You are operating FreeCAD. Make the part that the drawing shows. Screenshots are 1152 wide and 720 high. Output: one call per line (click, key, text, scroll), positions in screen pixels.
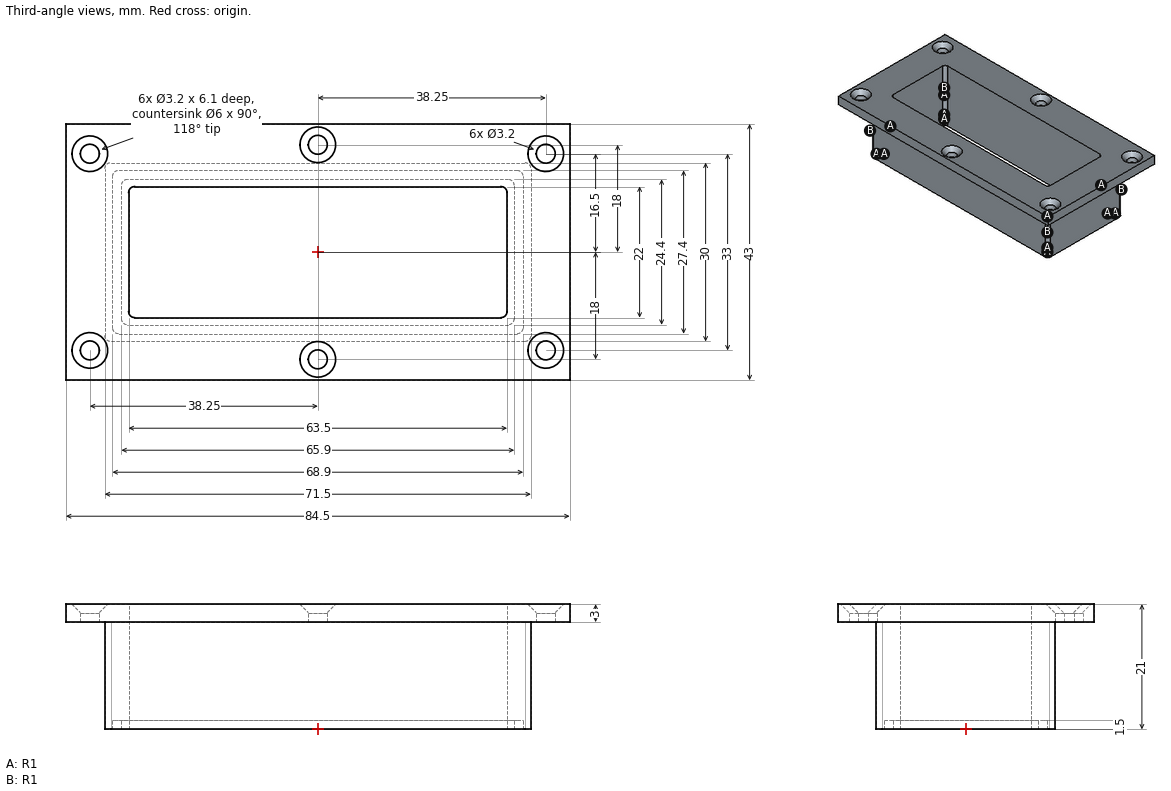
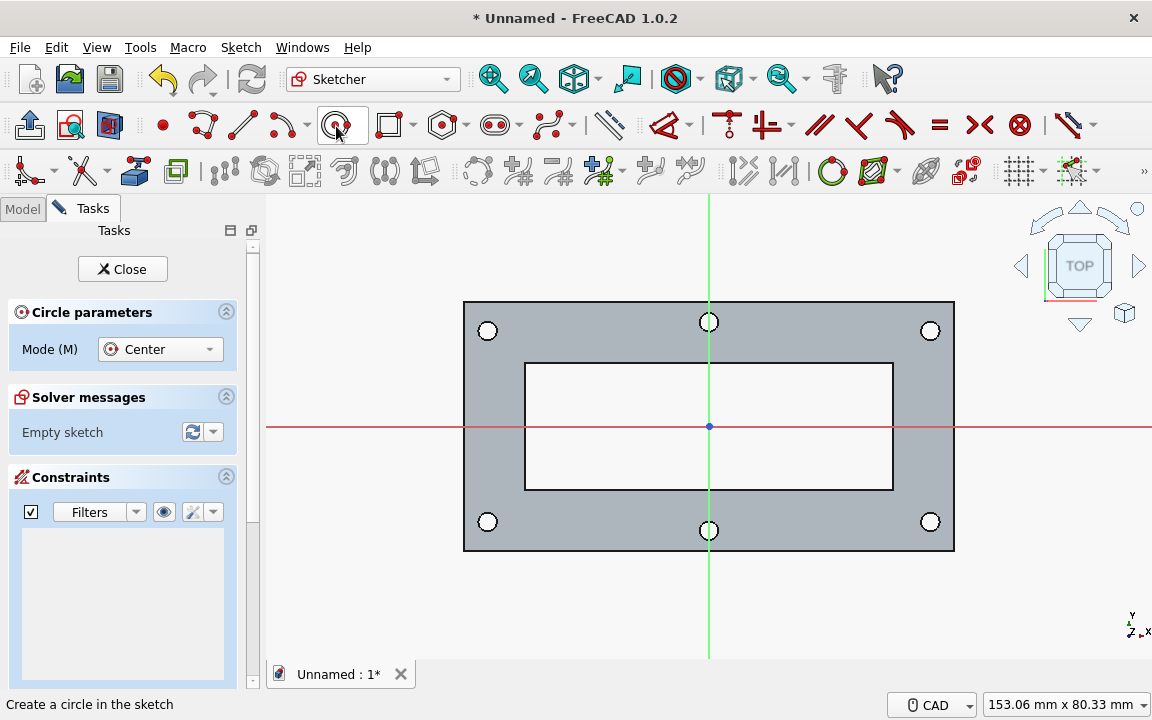
scroll(488, 331, up, 5)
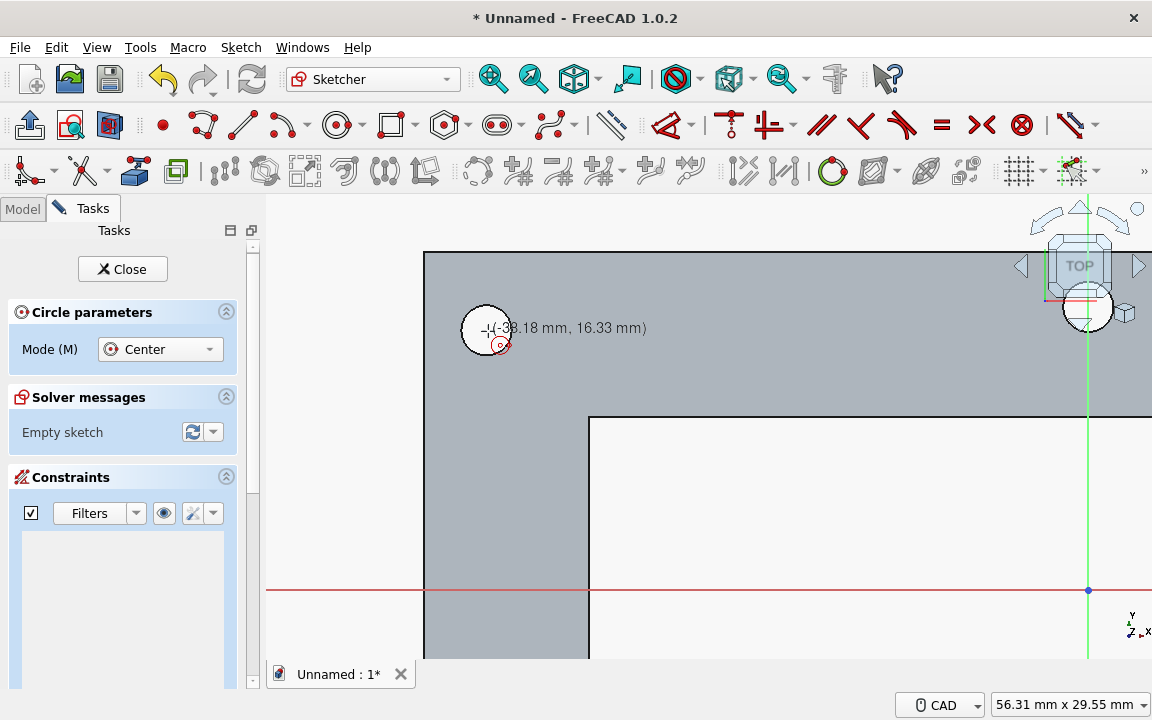
click(486, 330)
click(504, 313)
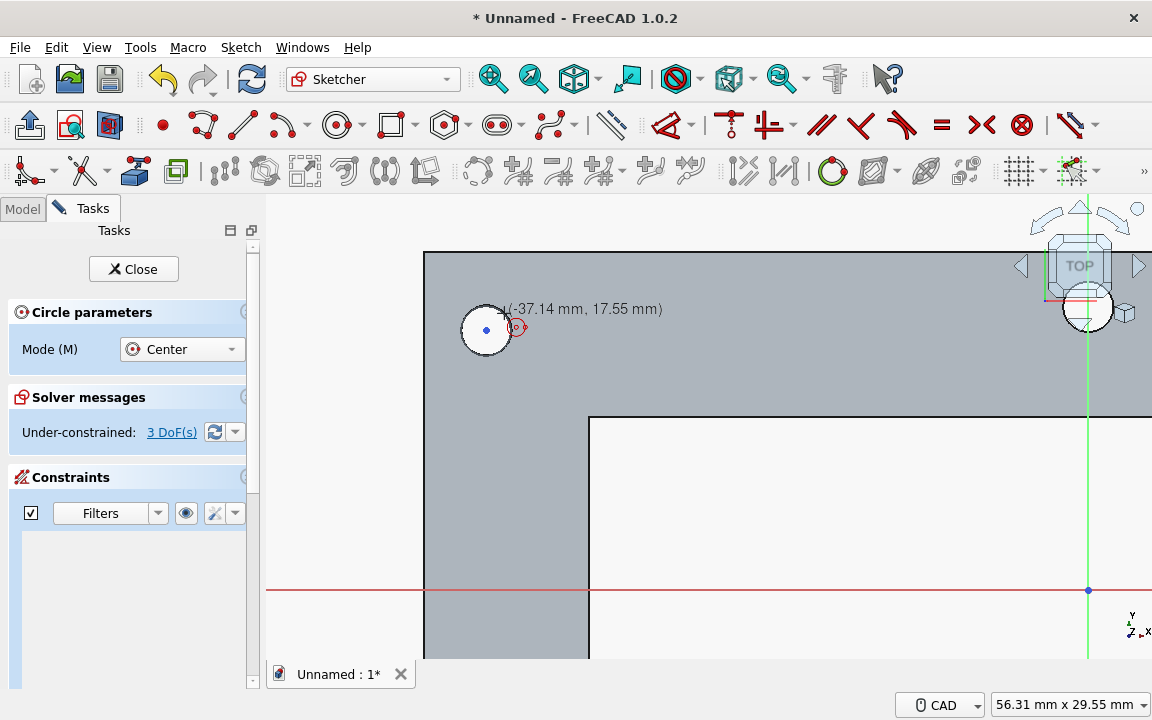
scroll(380, 331, down, 5)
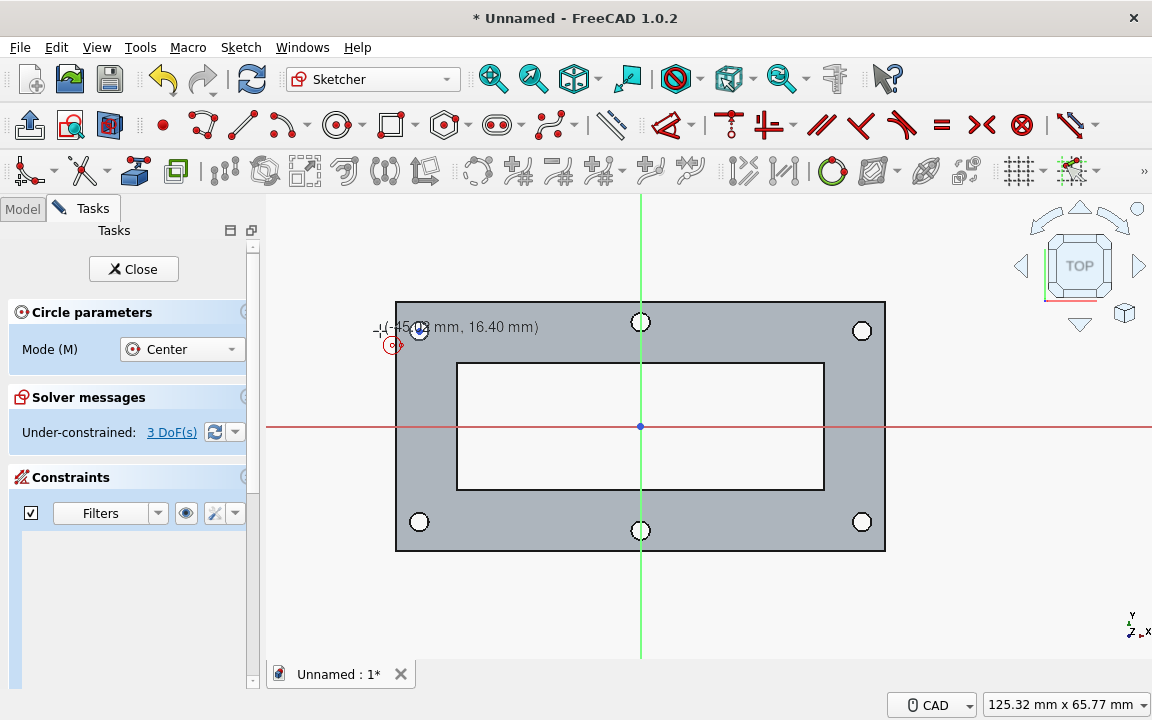
scroll(419, 522, up, 5)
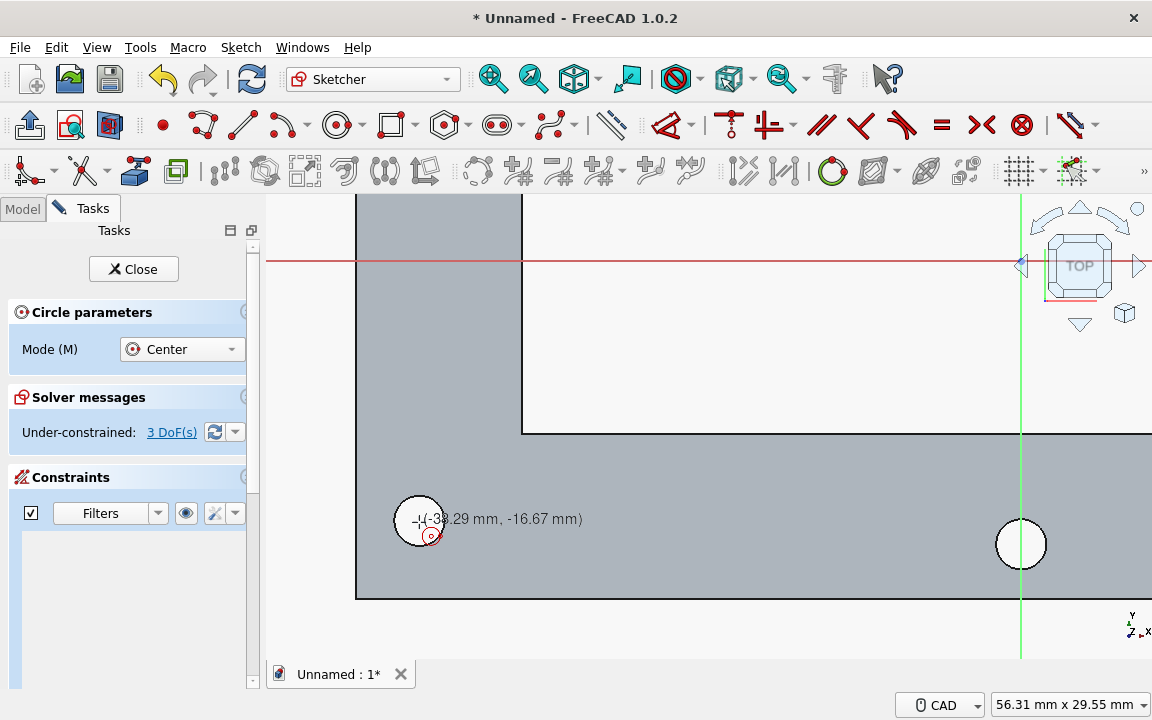
click(419, 521)
click(437, 503)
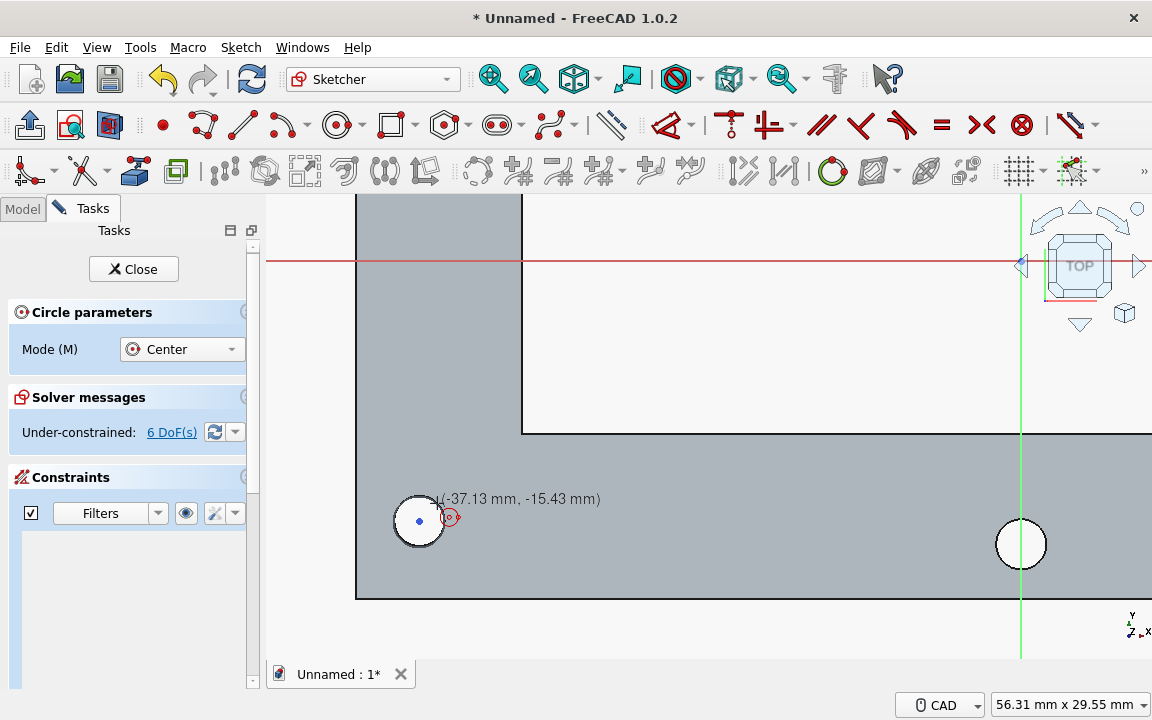
scroll(419, 523, down, 5)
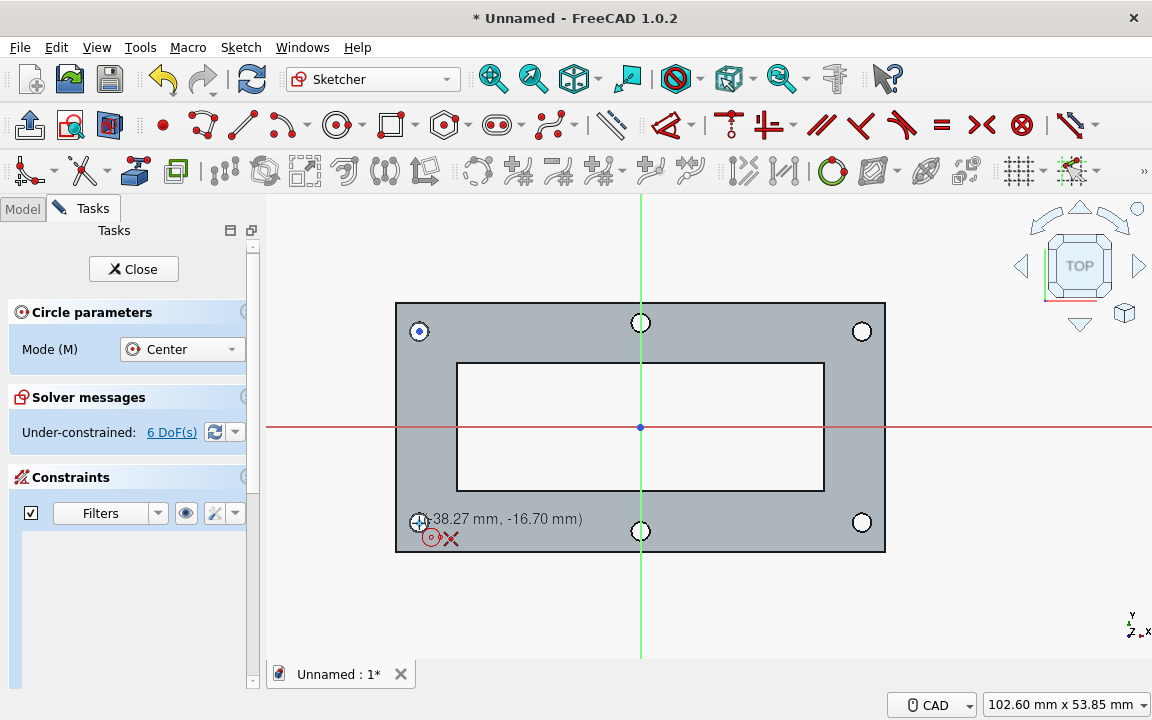
scroll(862, 332, up, 5)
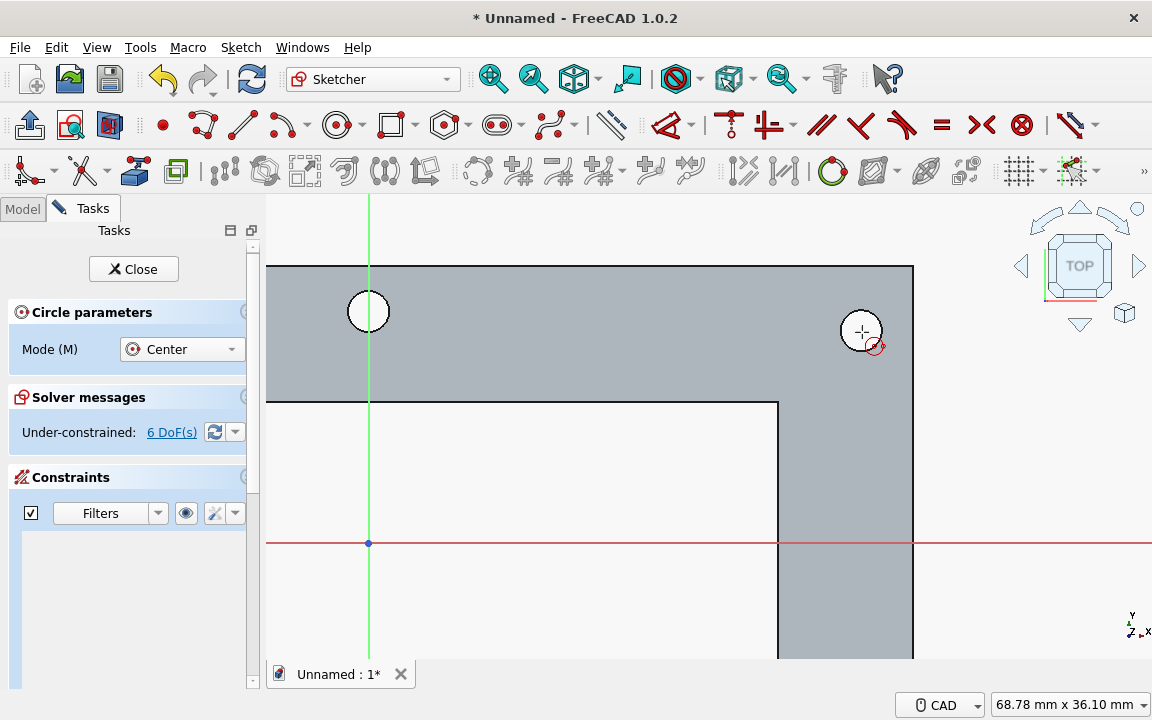
click(861, 330)
click(879, 313)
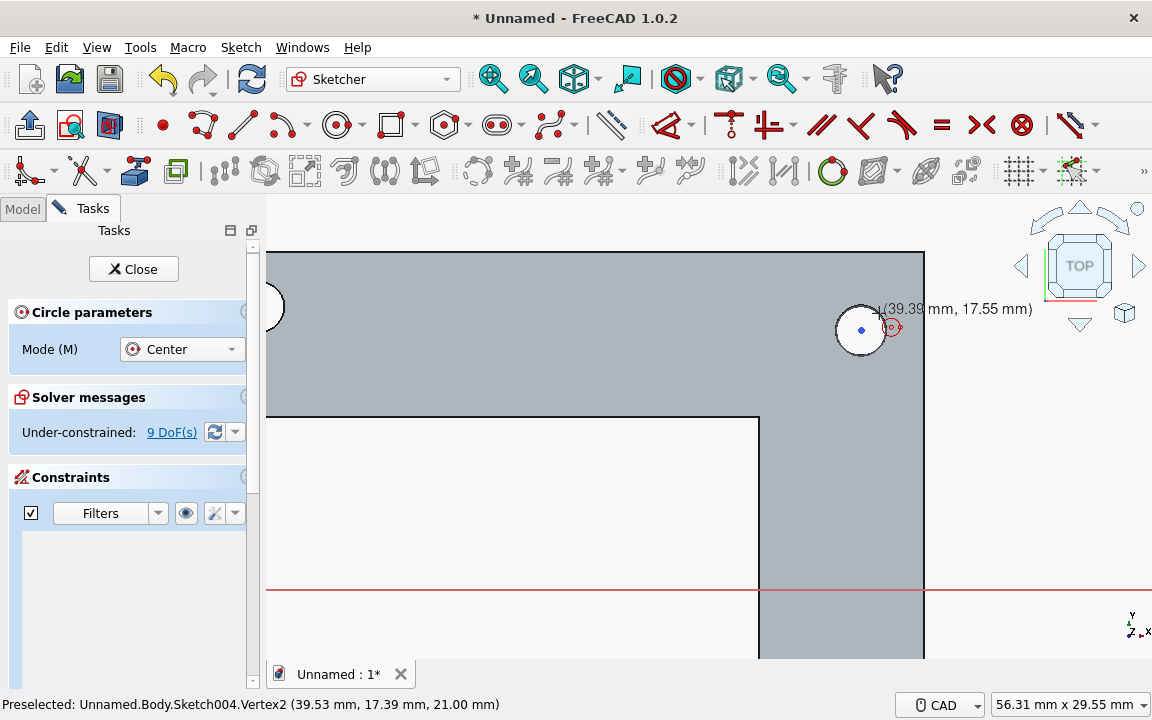
scroll(862, 331, down, 5)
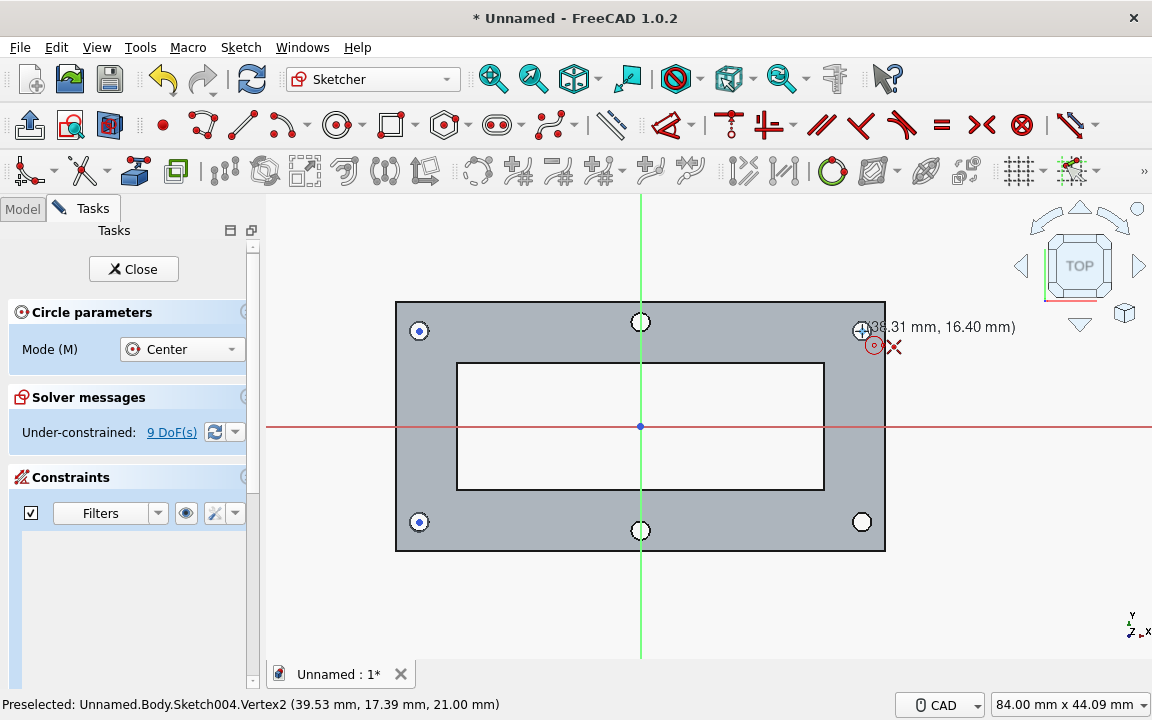
scroll(862, 522, up, 5)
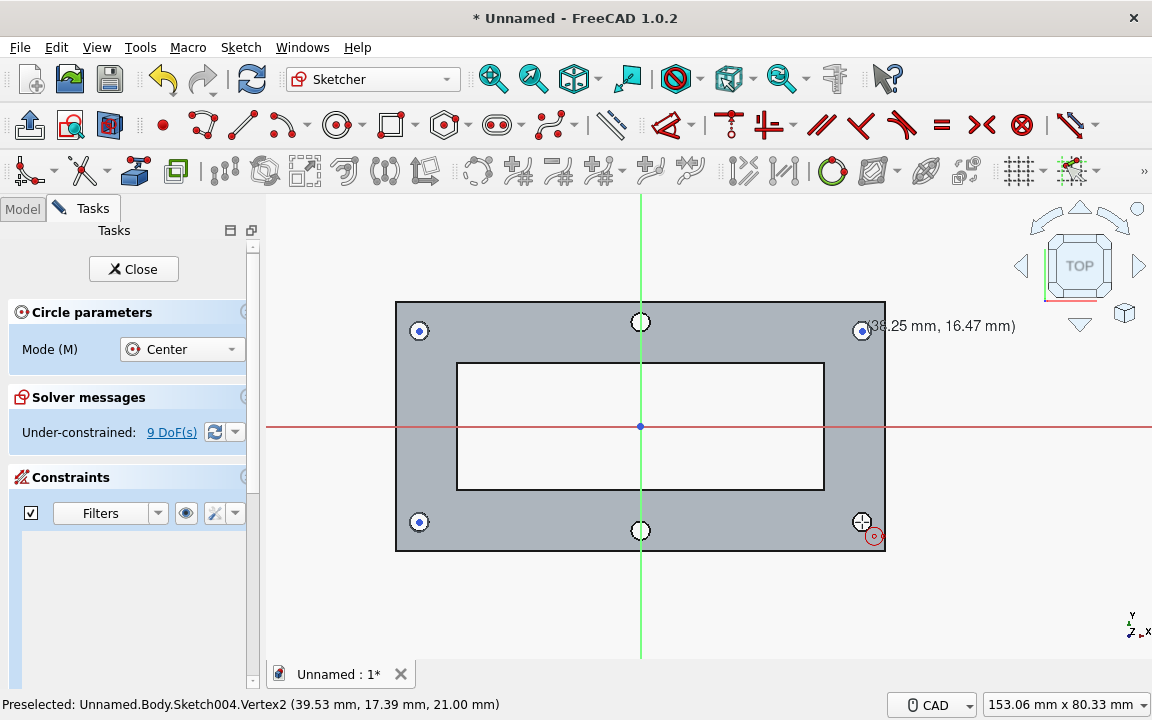
click(861, 521)
click(879, 503)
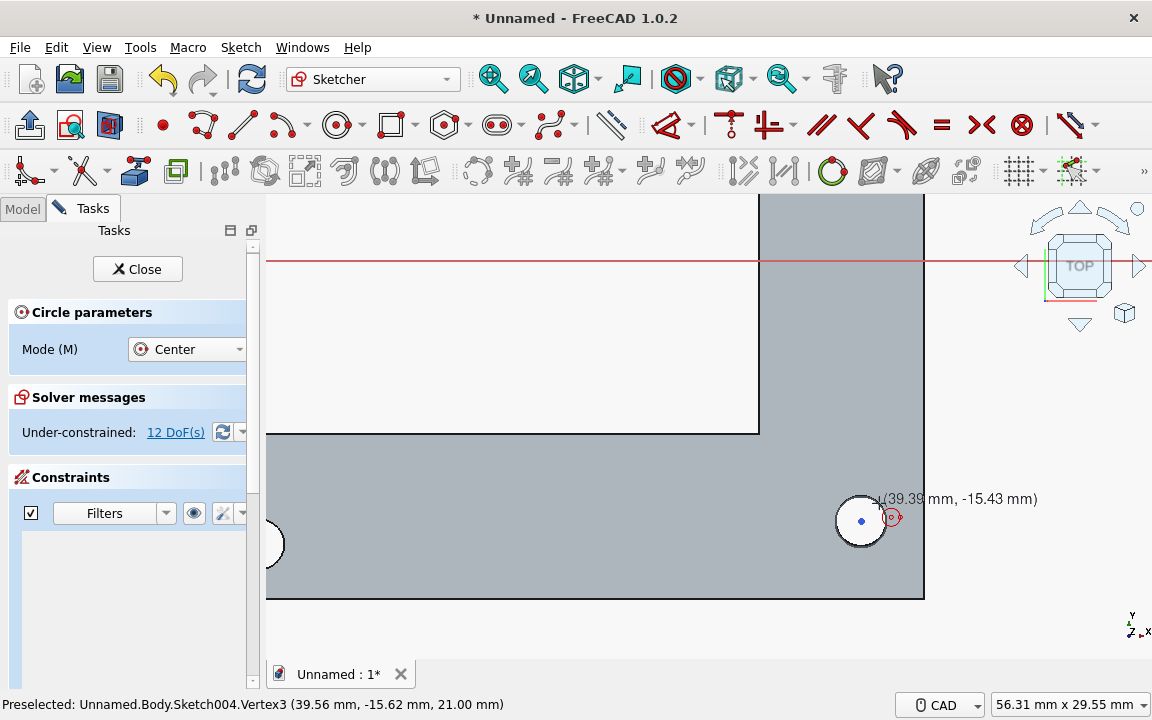
scroll(862, 523, down, 5)